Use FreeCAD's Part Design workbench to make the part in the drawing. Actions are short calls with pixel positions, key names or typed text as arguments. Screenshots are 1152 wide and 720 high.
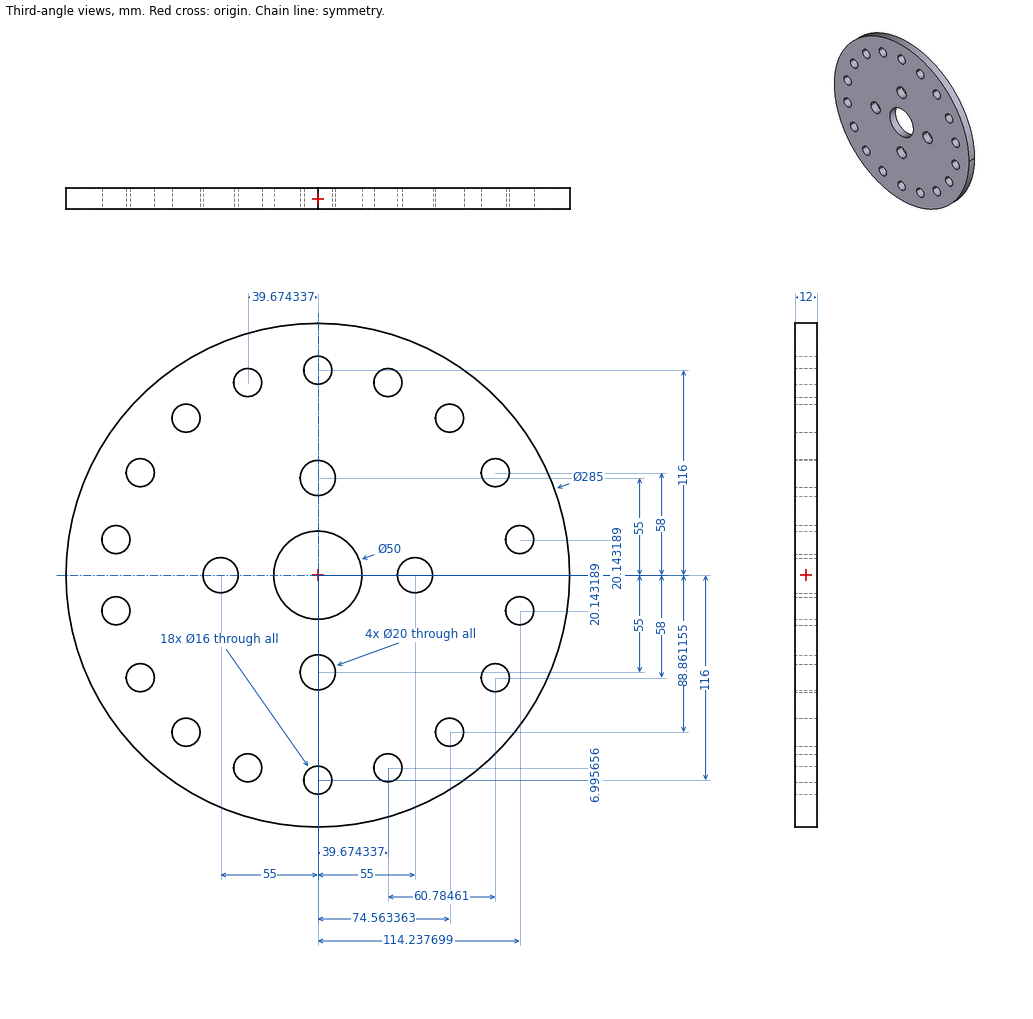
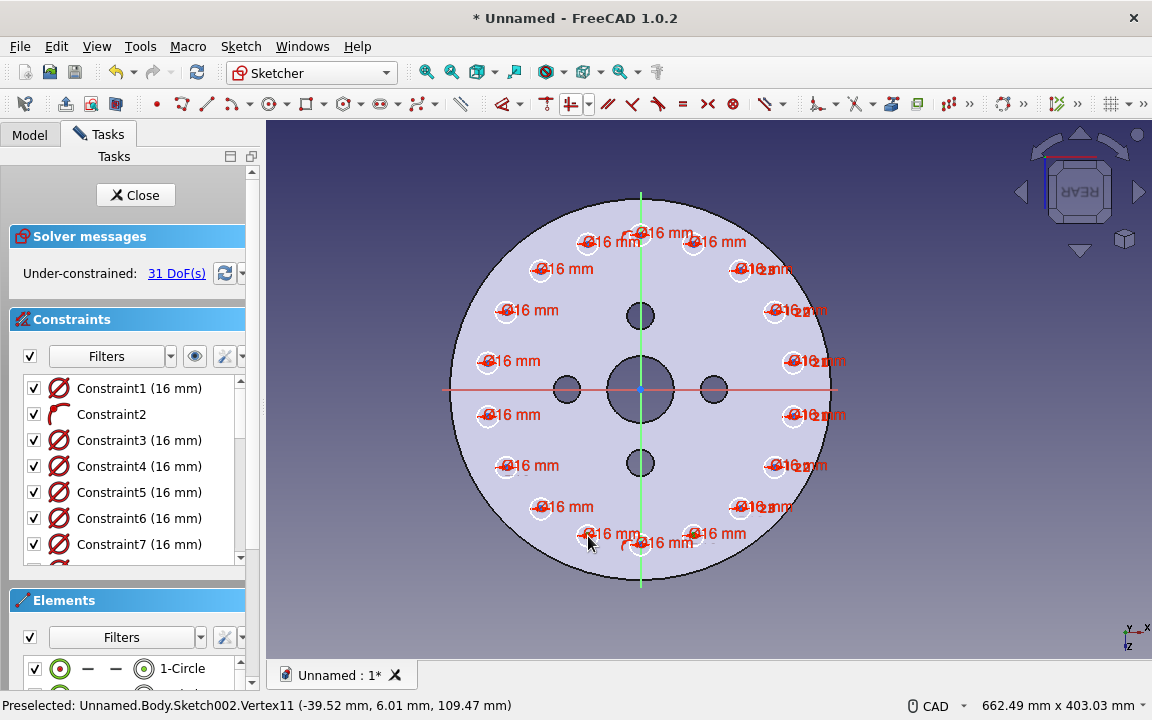
click(588, 104)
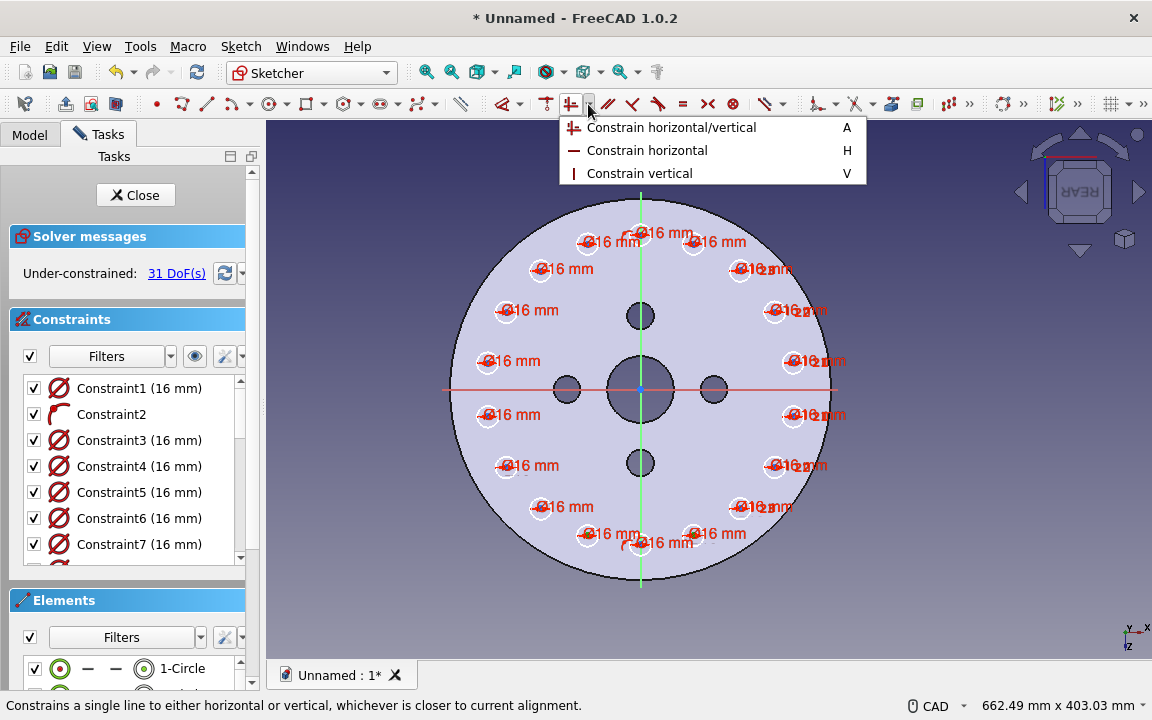
click(713, 150)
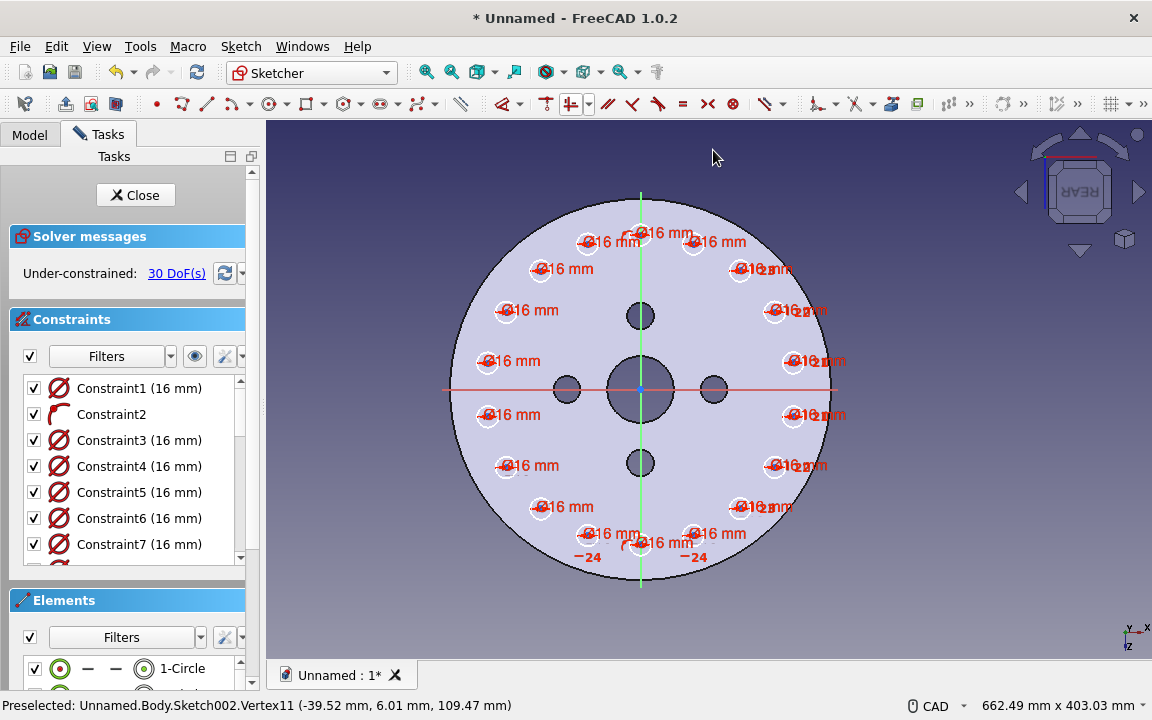
click(740, 509)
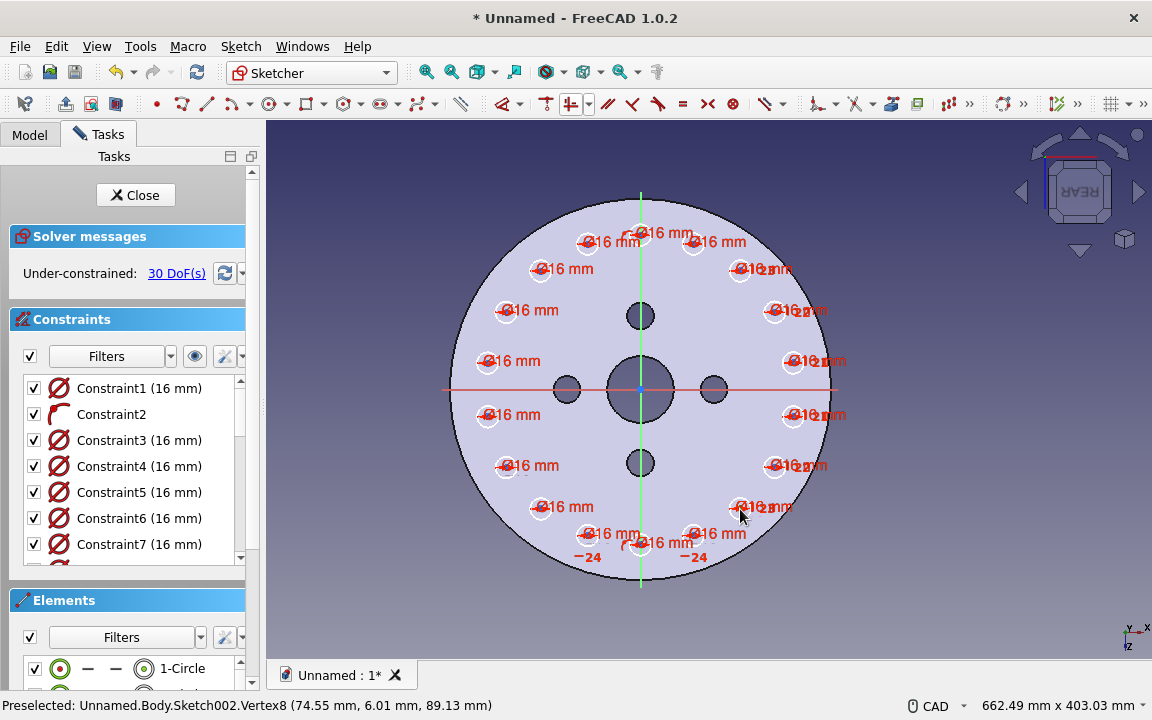
click(541, 509)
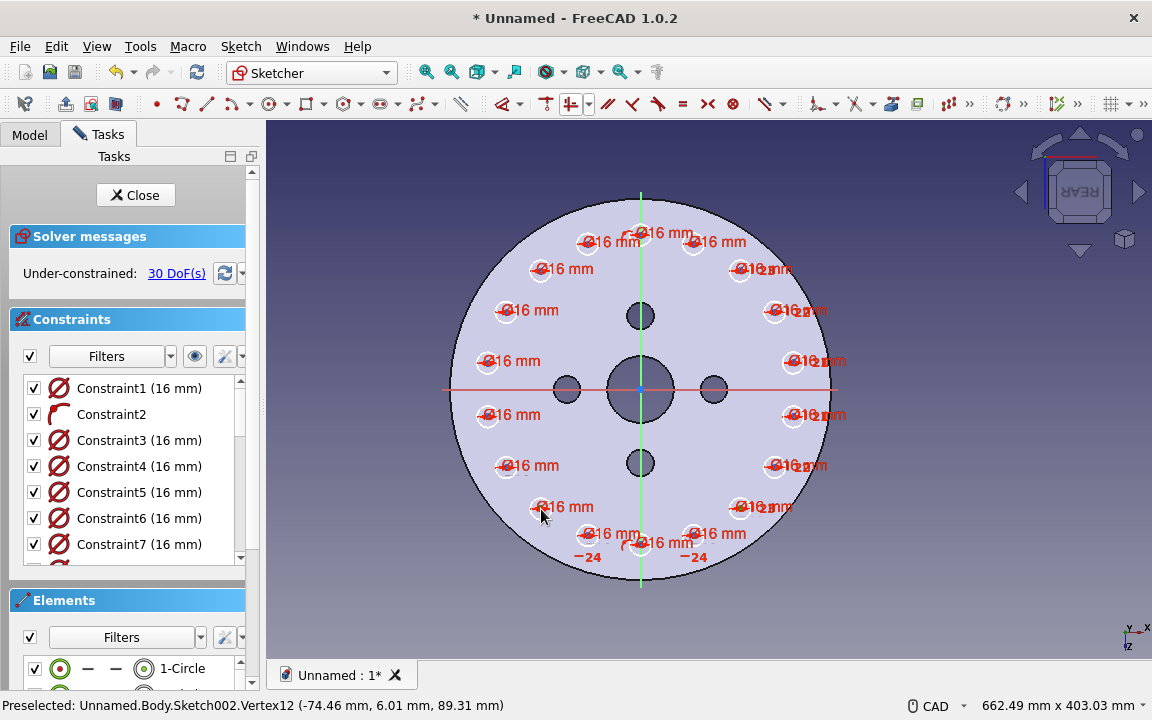
key(h)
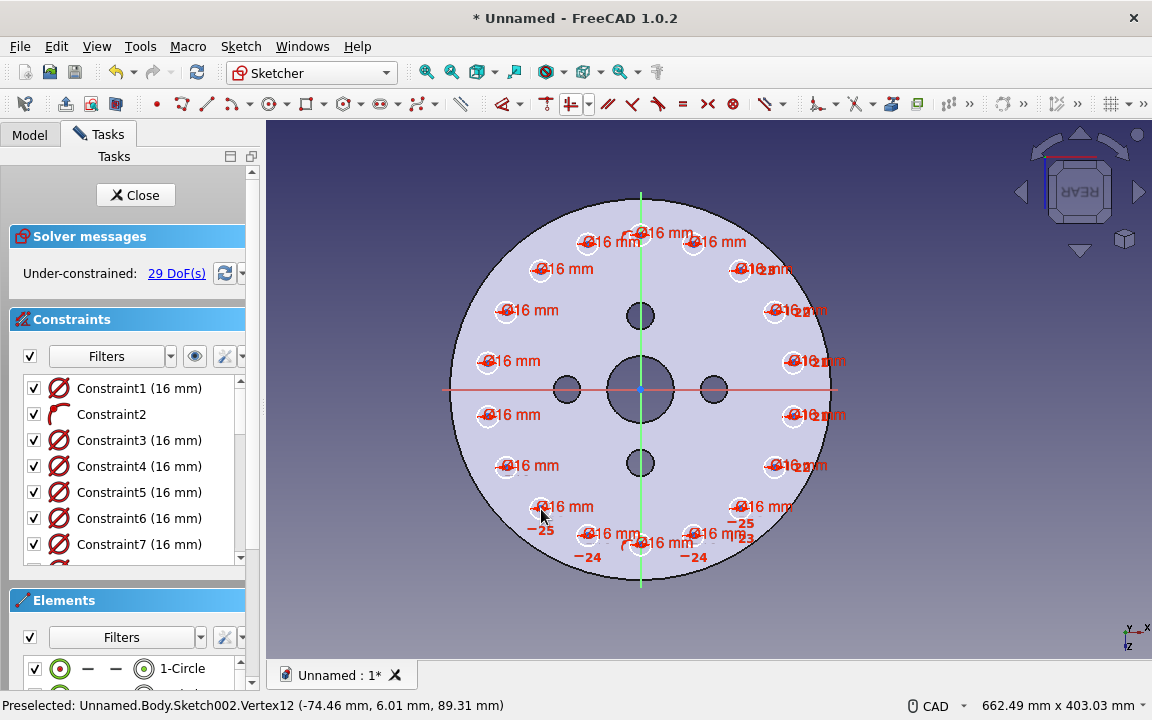
click(488, 417)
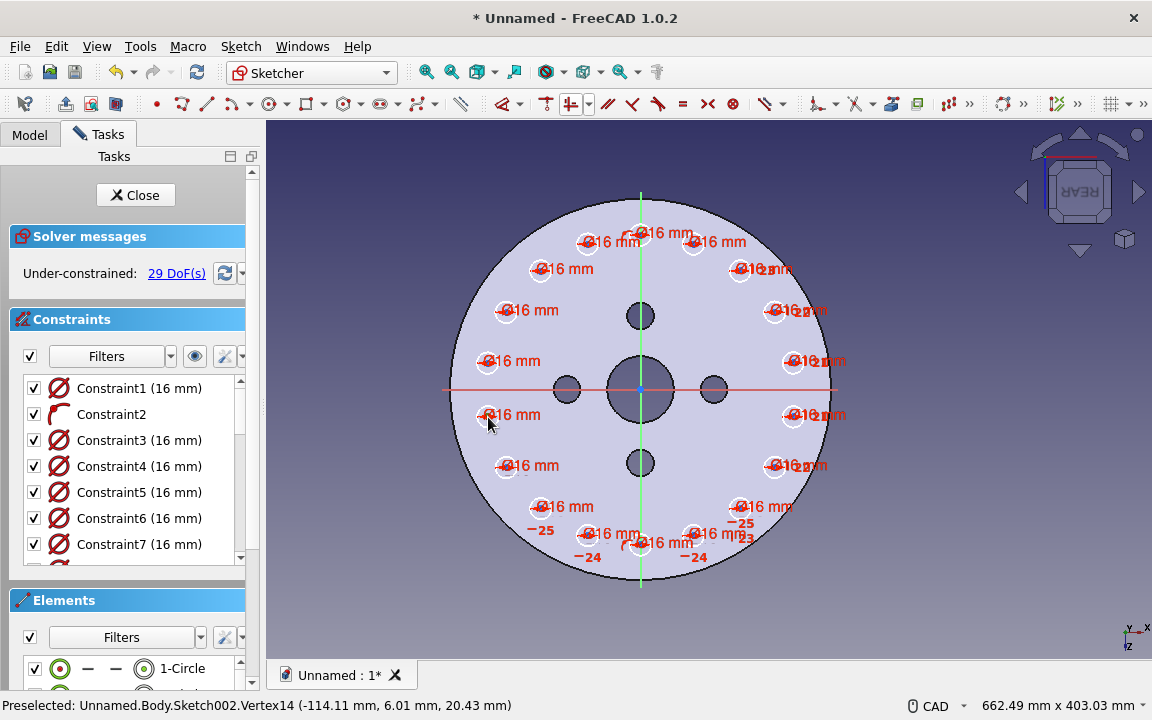
click(488, 363)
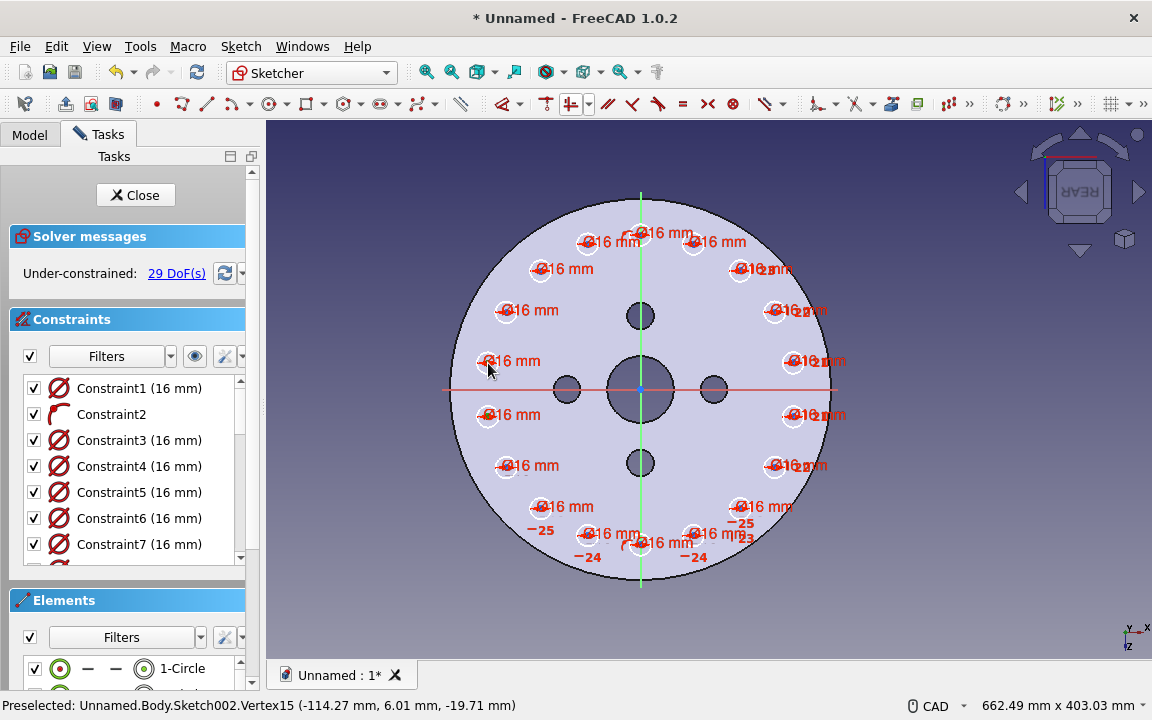
key(v)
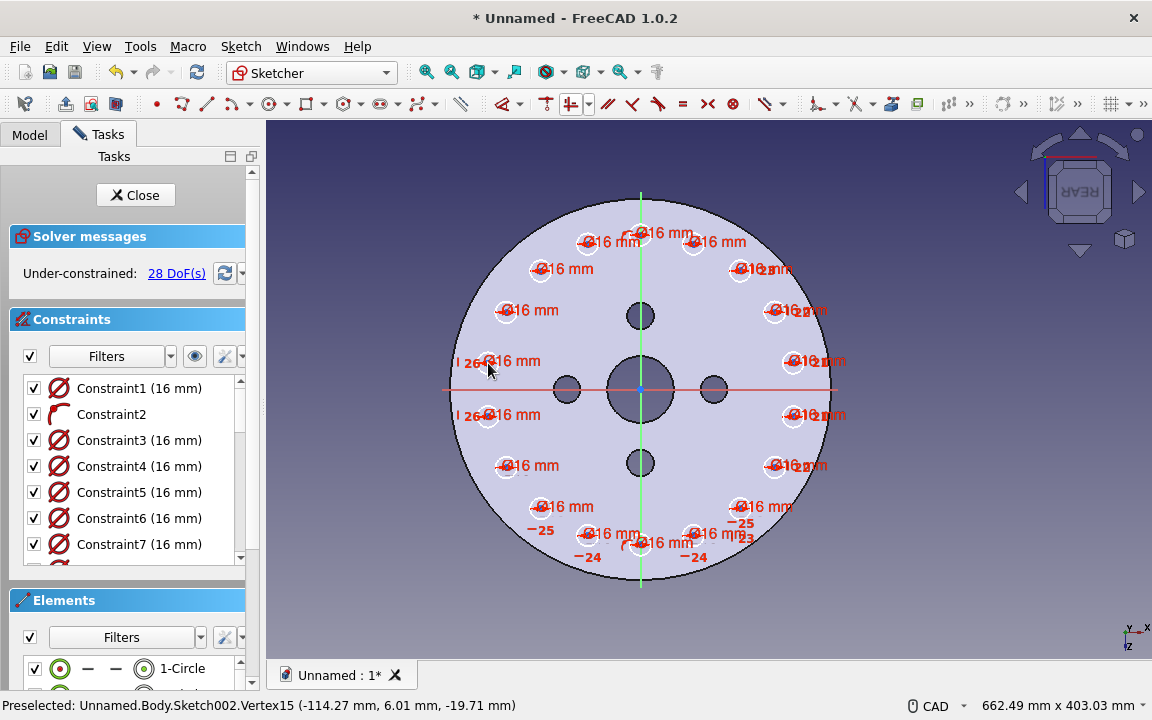
click(506, 468)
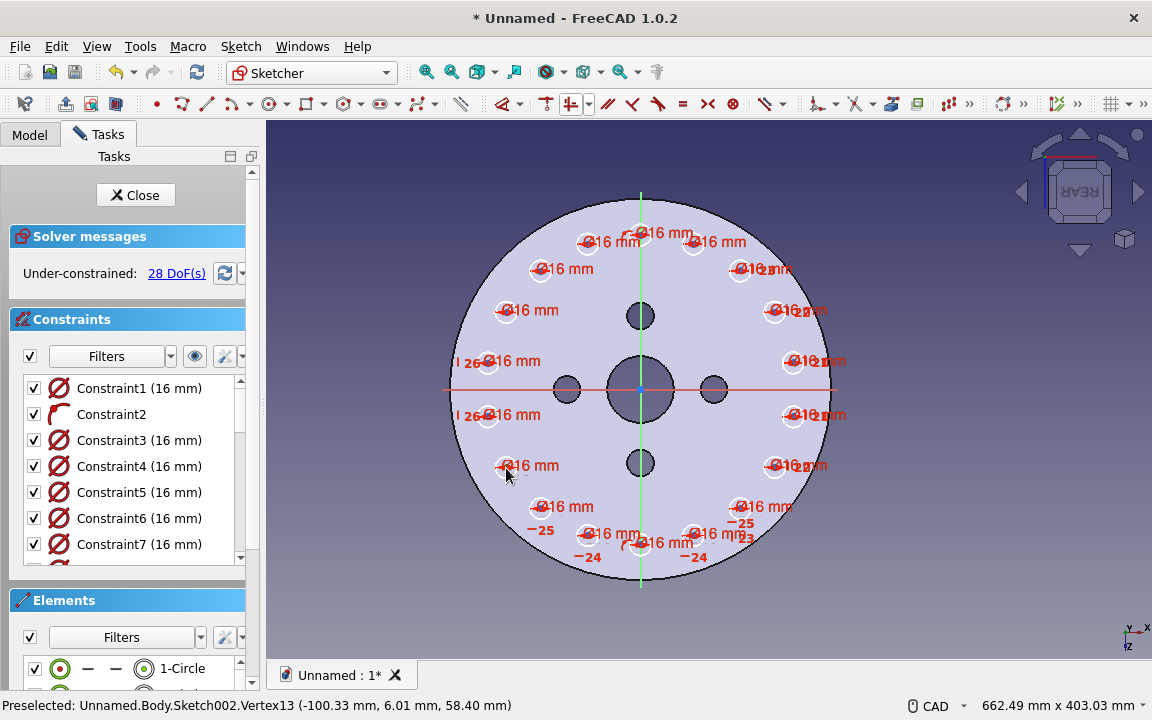
click(506, 312)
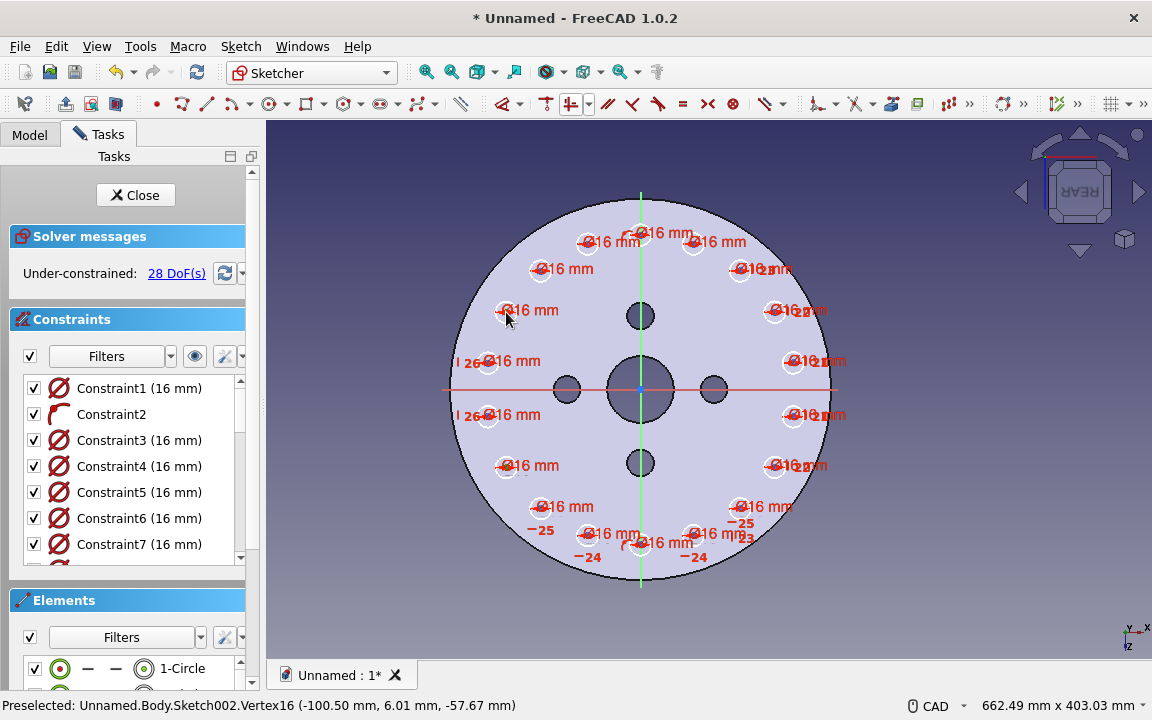
key(v)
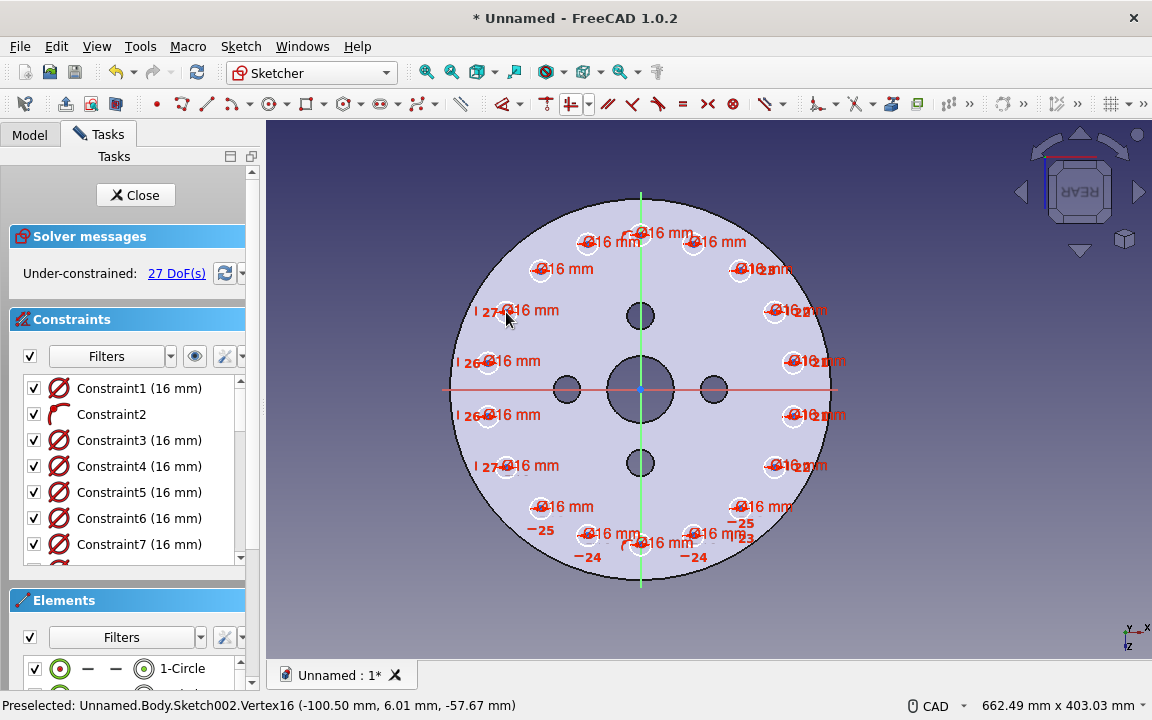
click(693, 244)